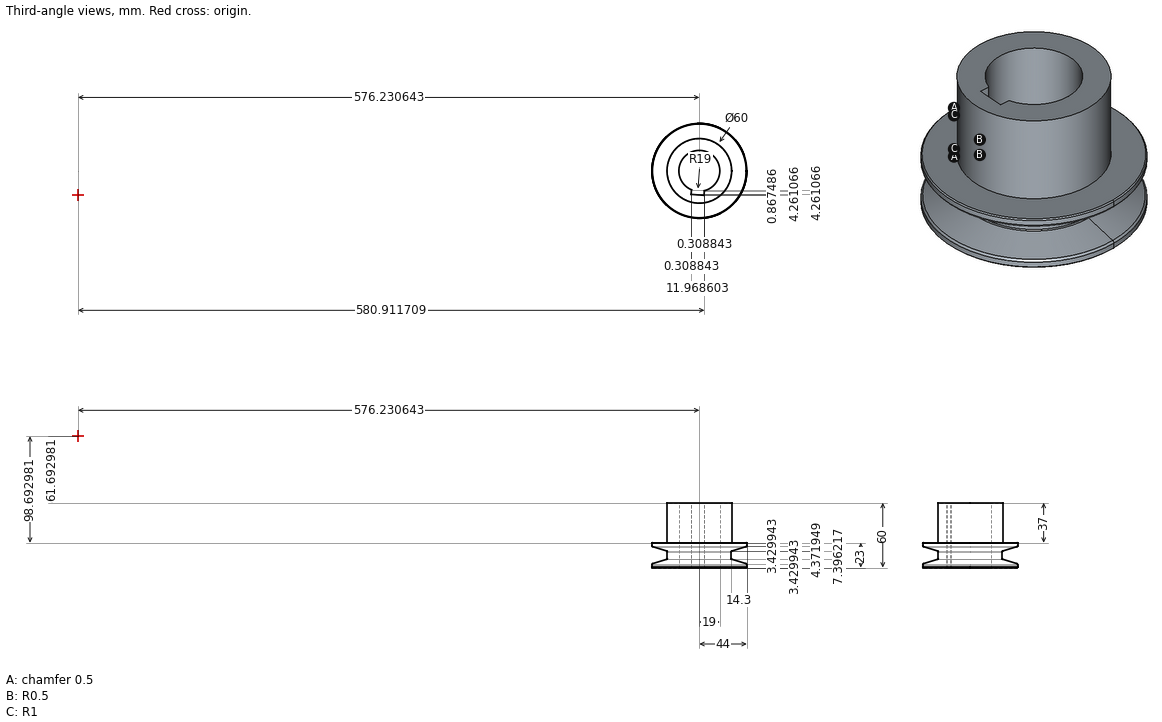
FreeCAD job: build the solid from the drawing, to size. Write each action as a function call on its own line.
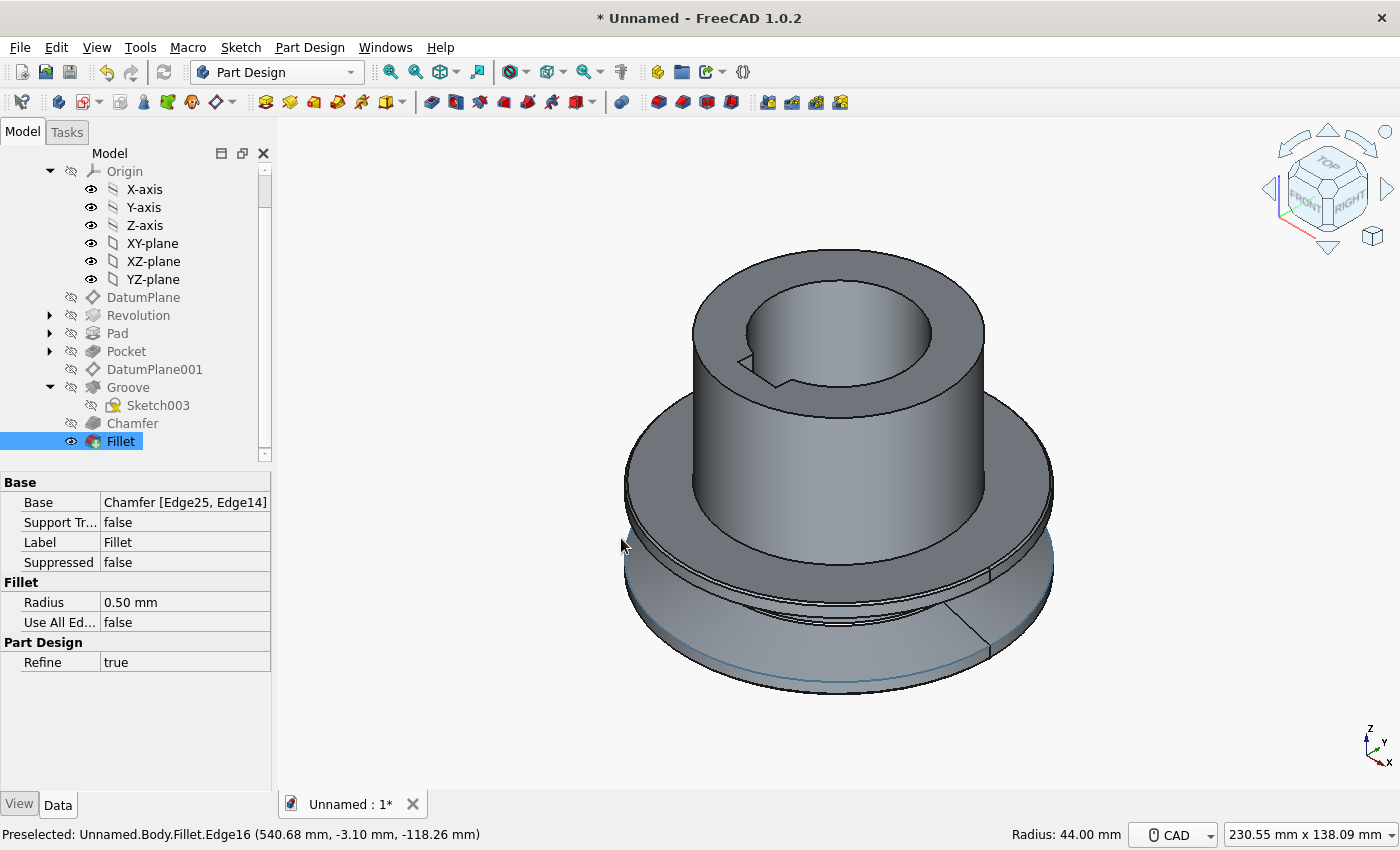
key(1)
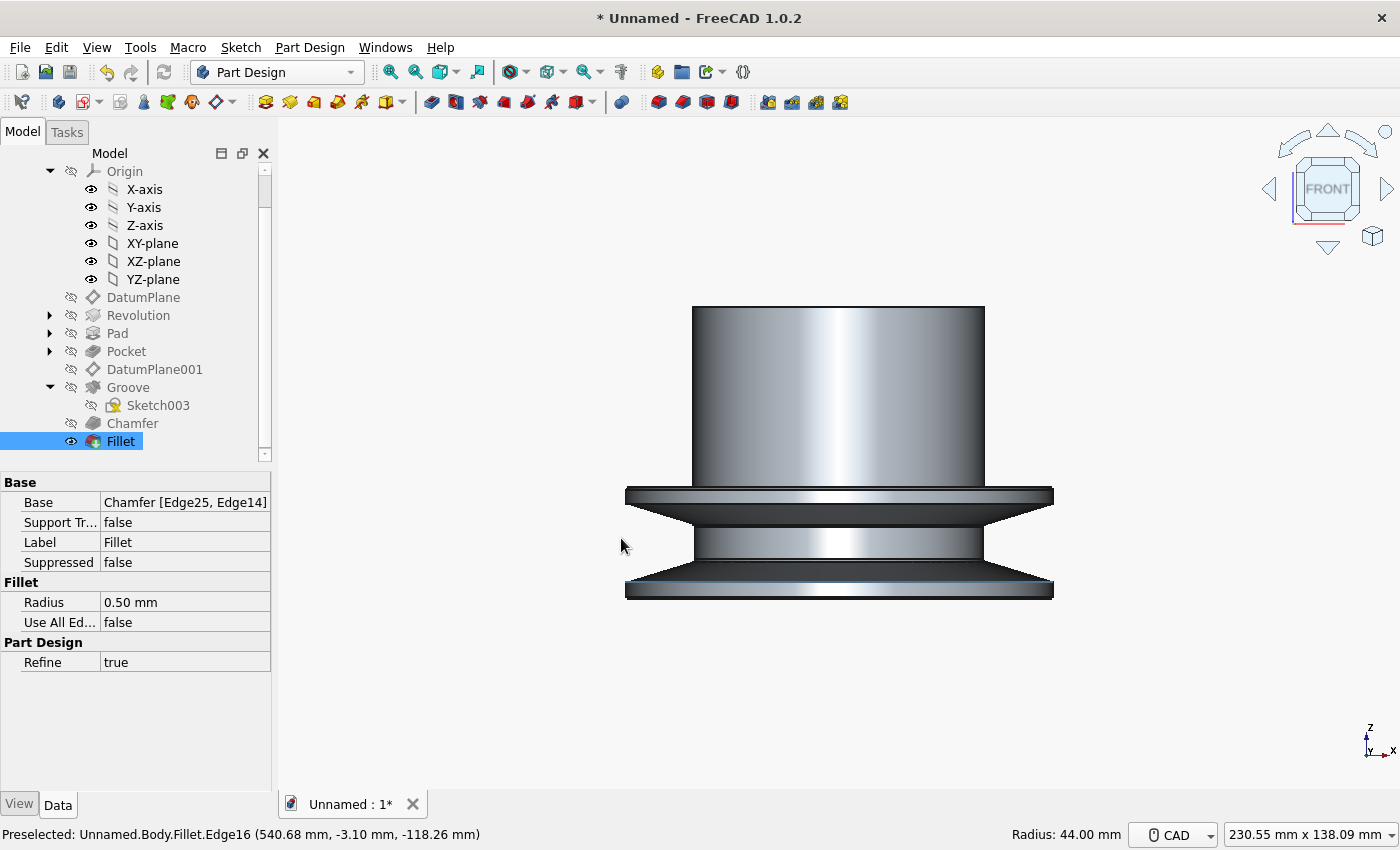
click(392, 72)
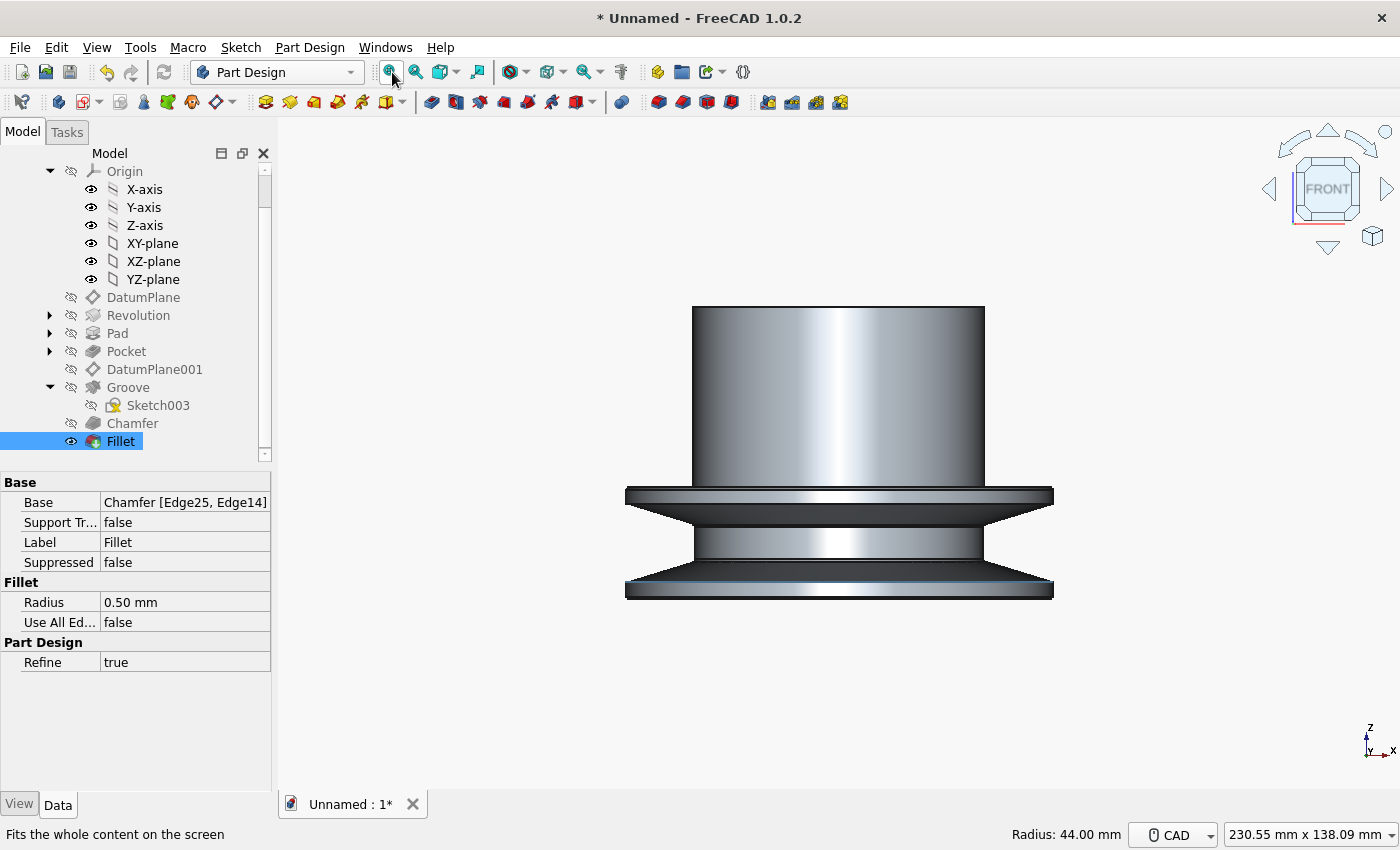
key(3)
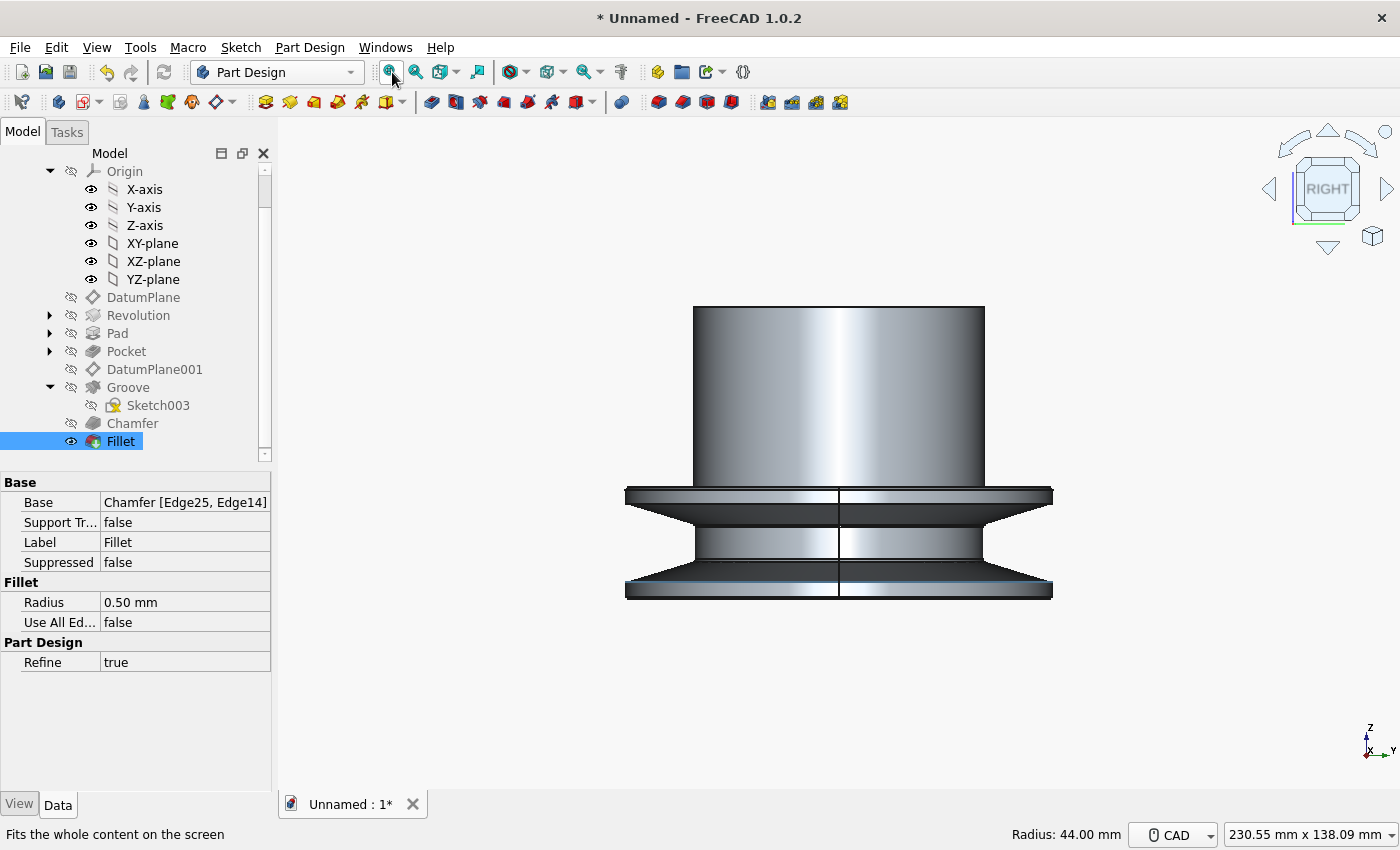
key(v)
key(f)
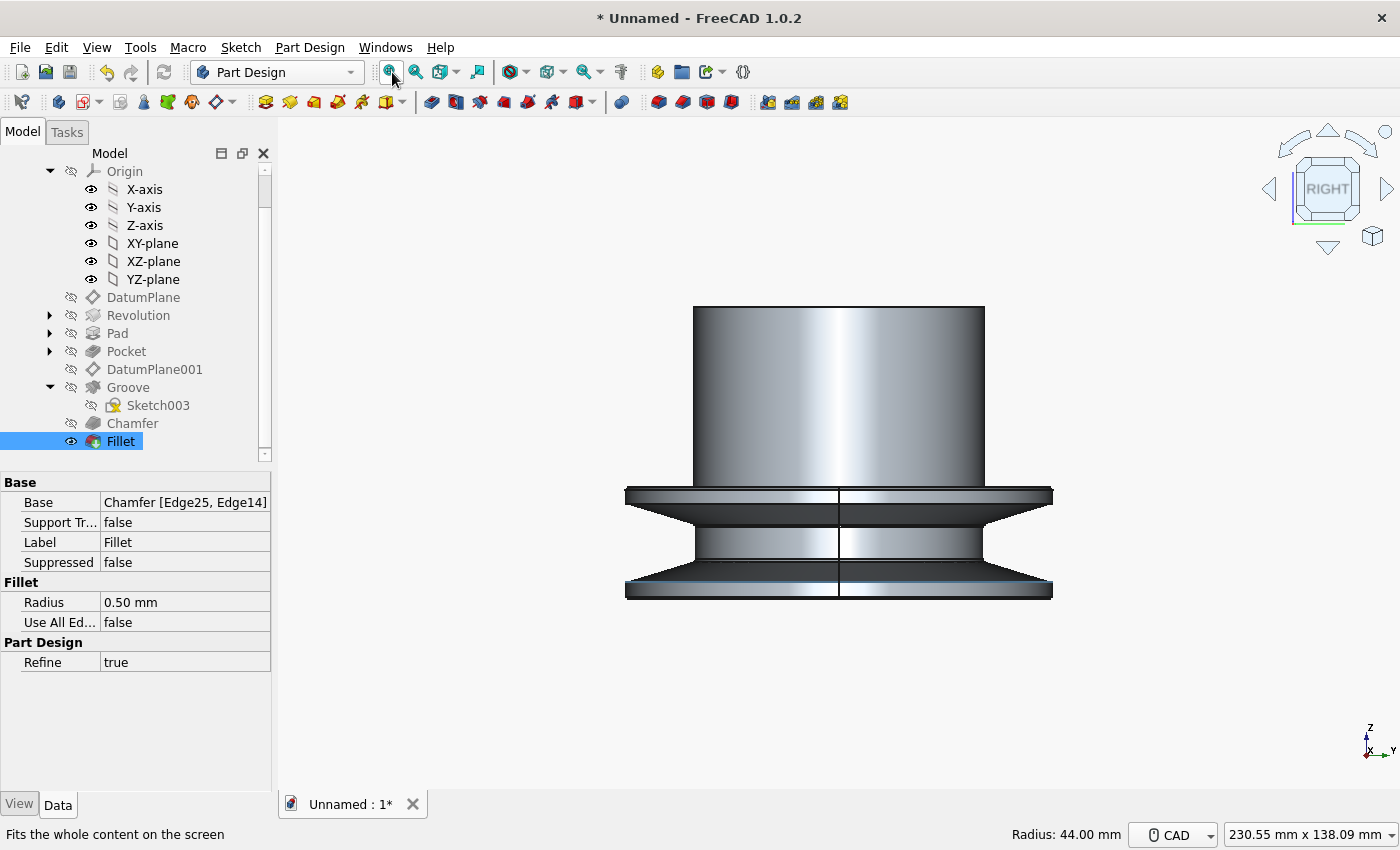
click(713, 503, ctrl)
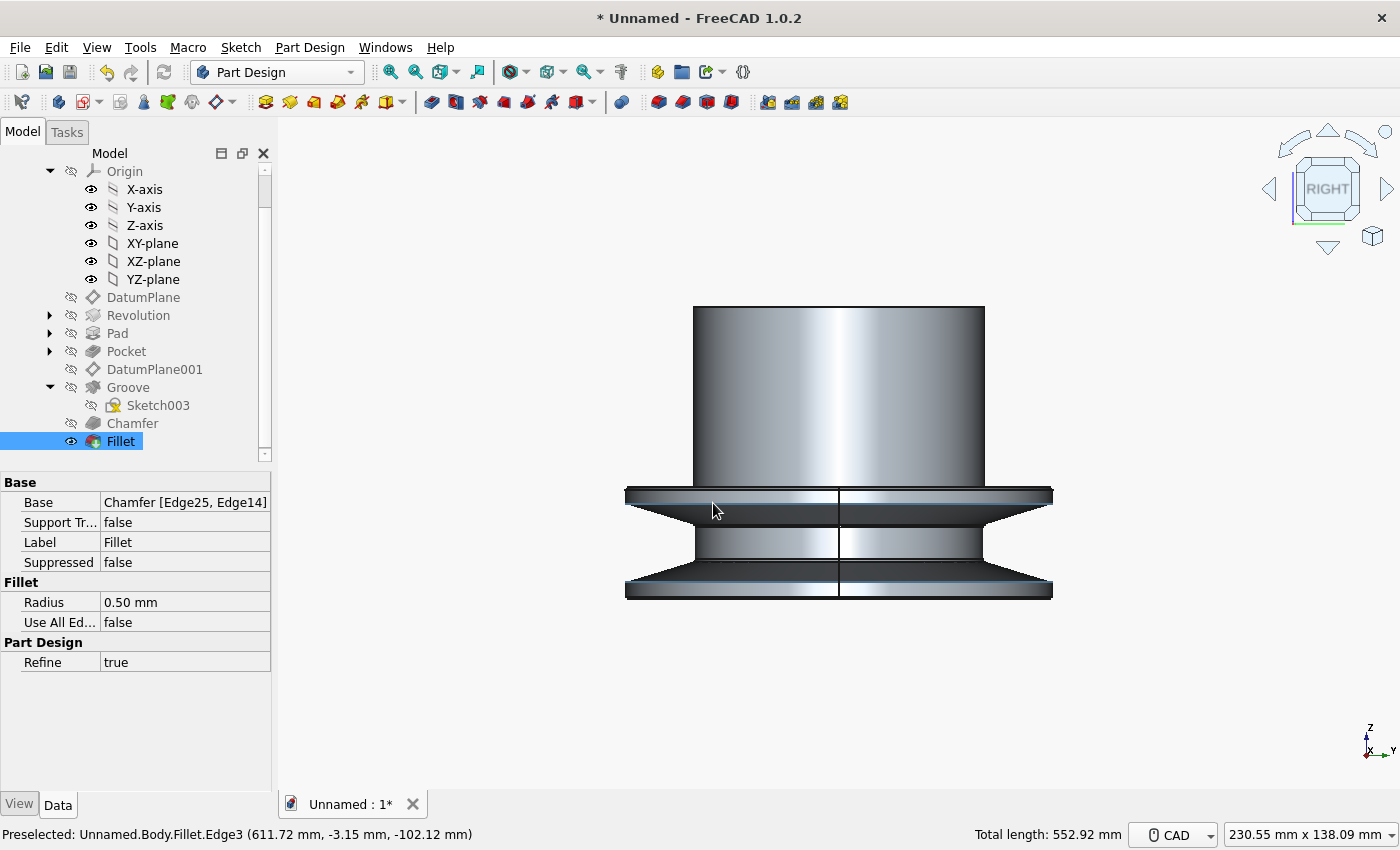
click(660, 102)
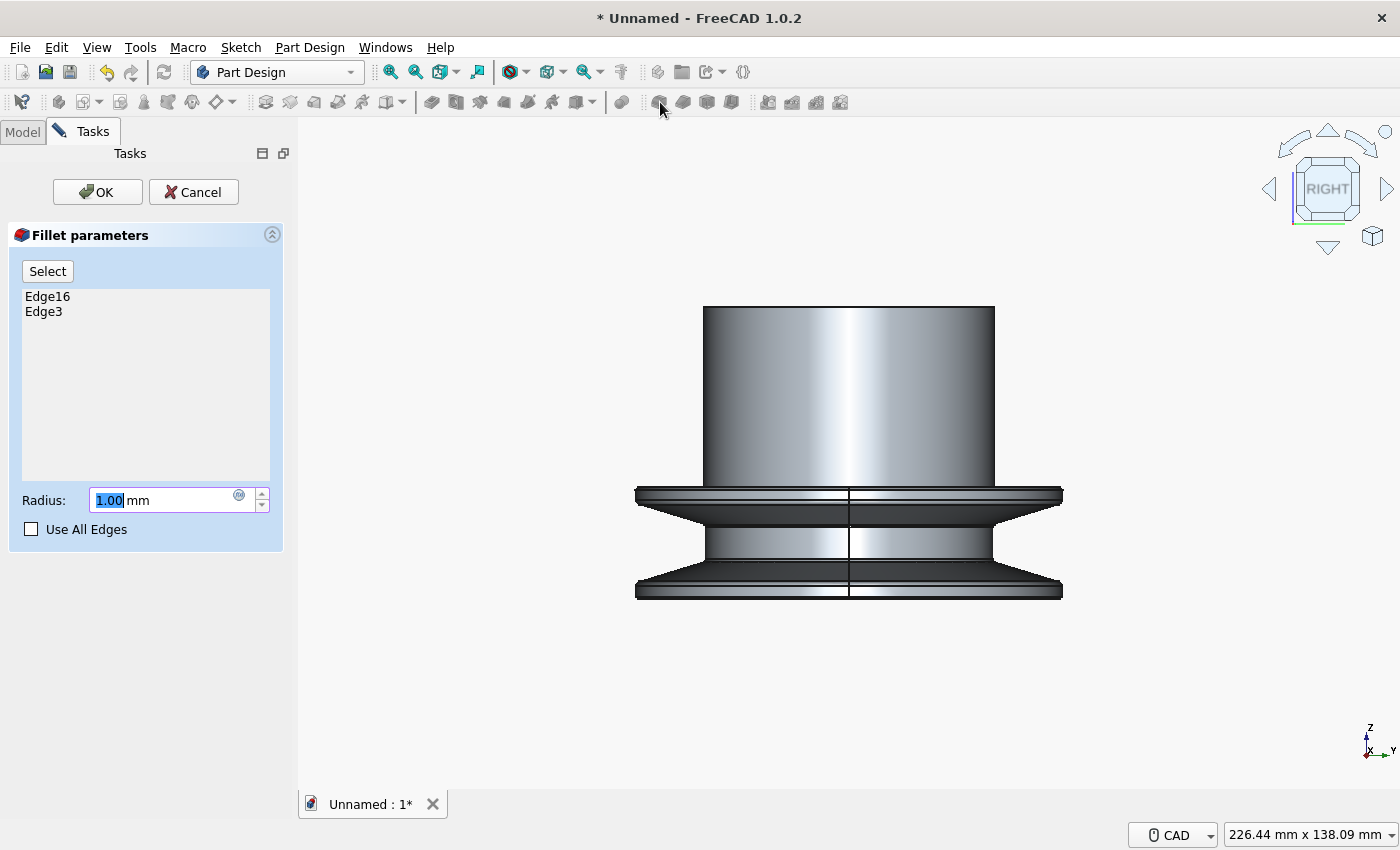
text(1)
key(Tab)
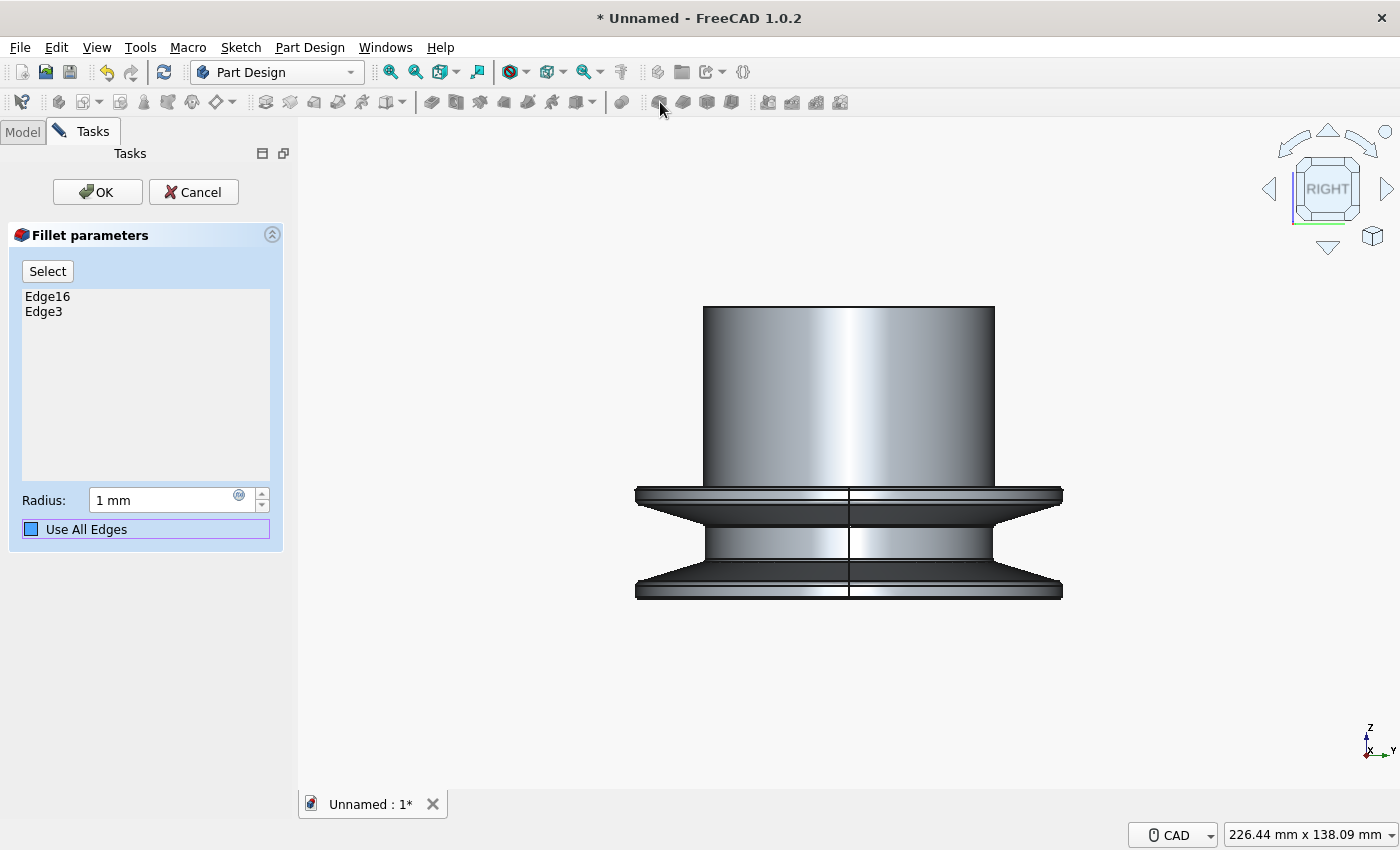
click(98, 192)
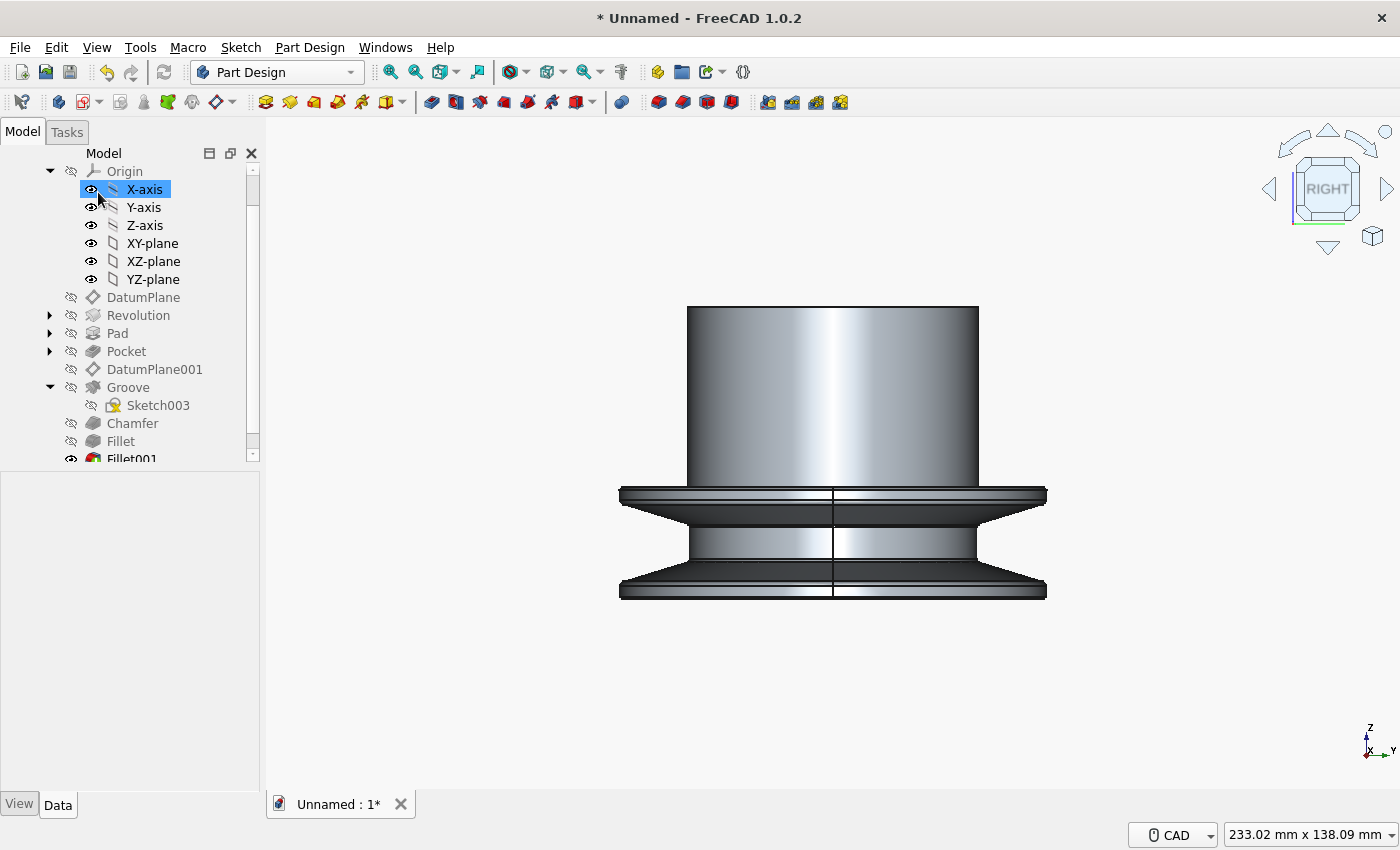
key(0)